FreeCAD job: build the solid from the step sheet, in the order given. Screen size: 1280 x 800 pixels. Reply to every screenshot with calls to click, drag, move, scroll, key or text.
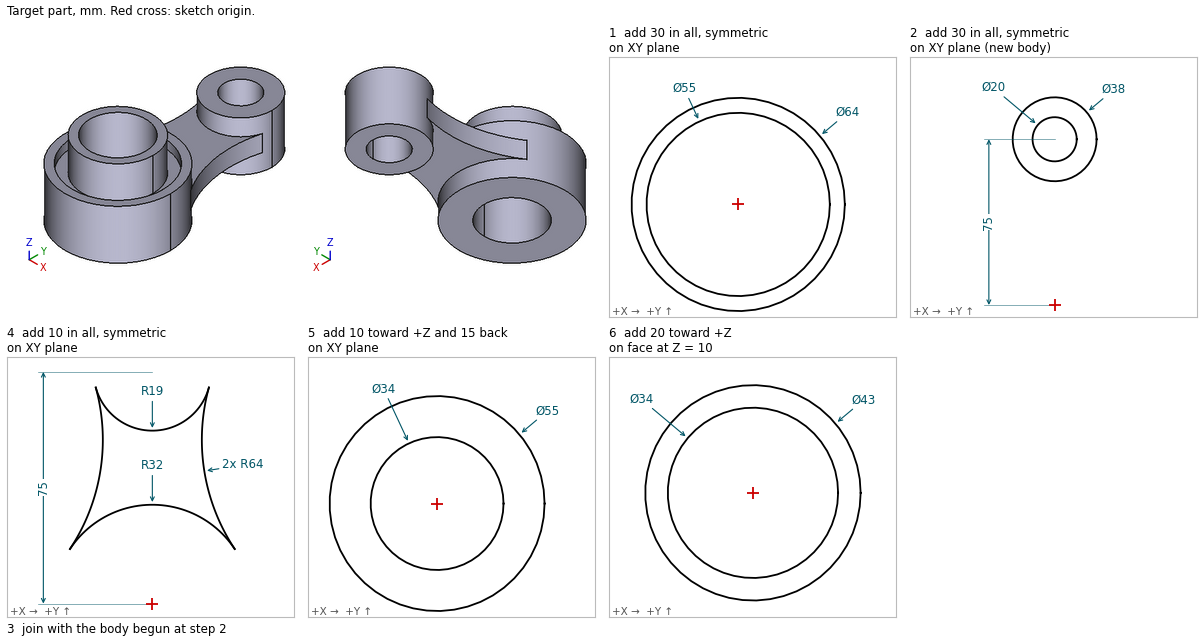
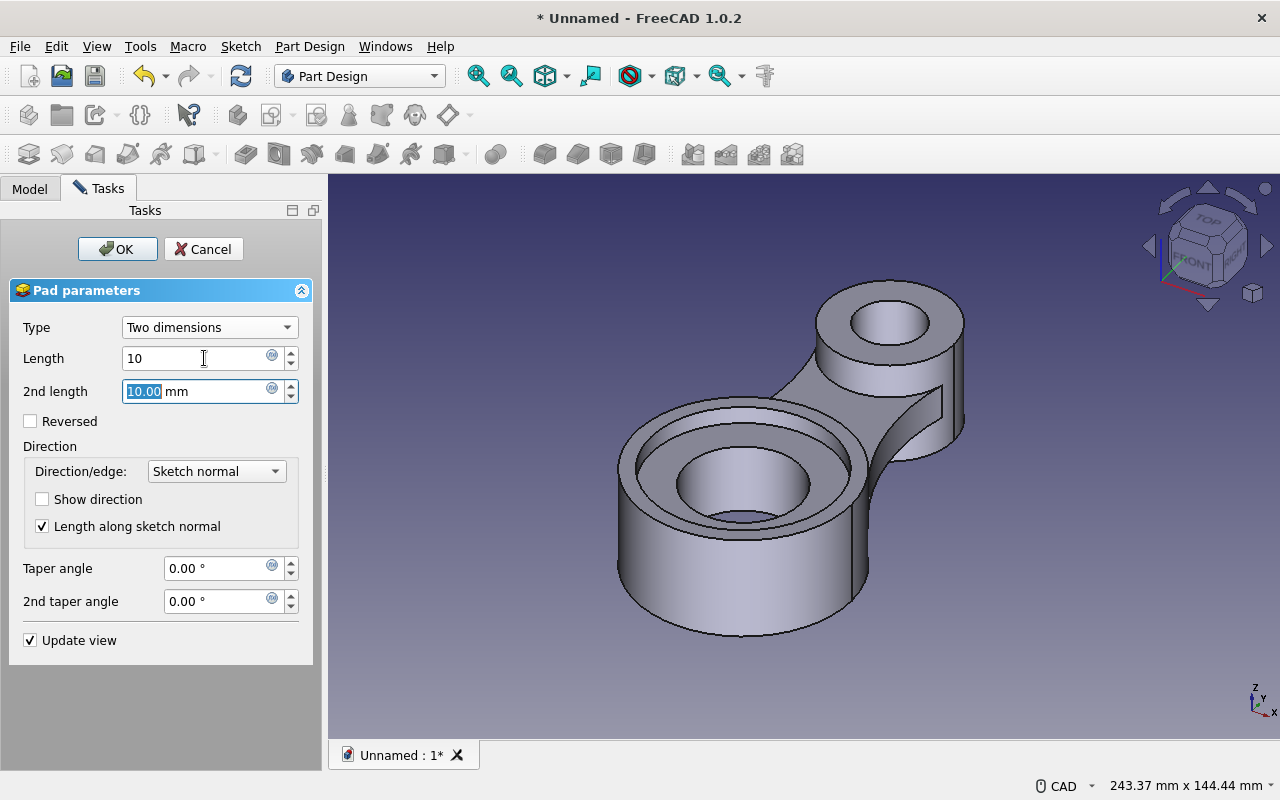
text(15)
key(Tab)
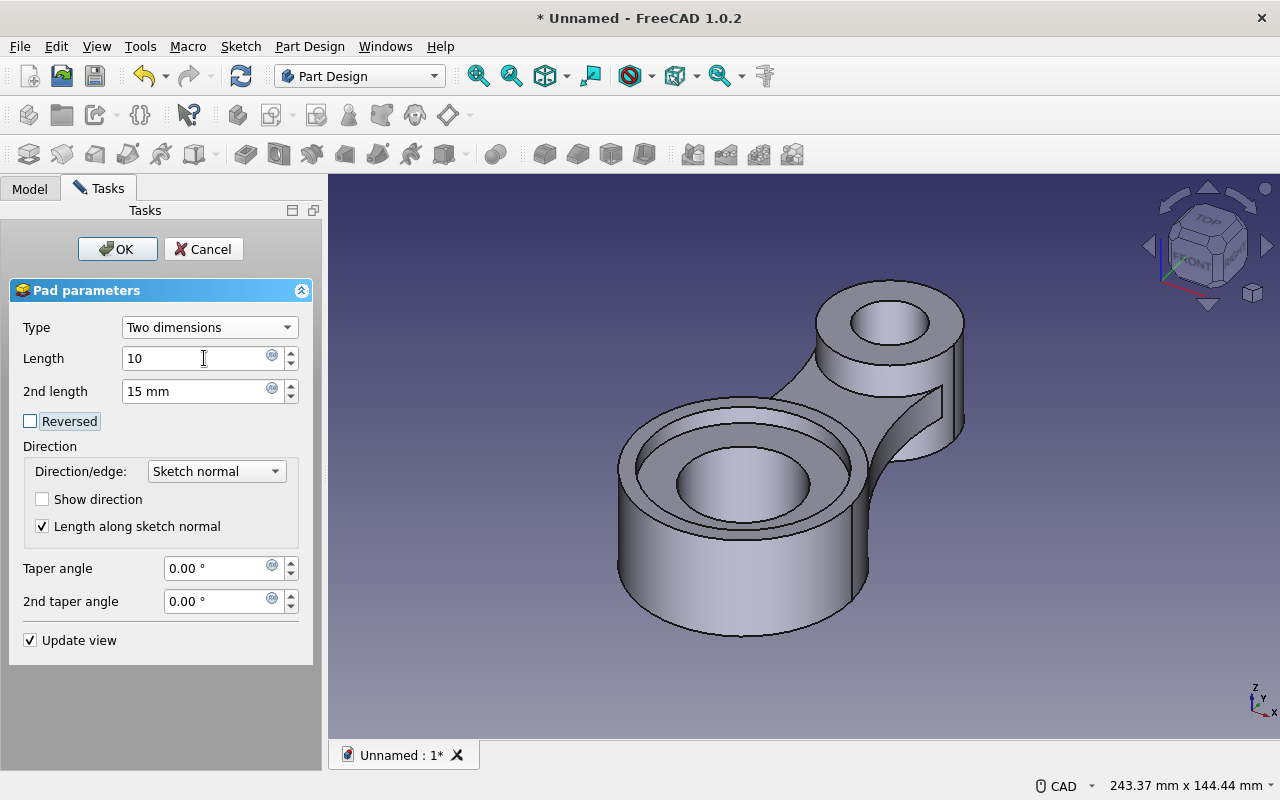
click(118, 249)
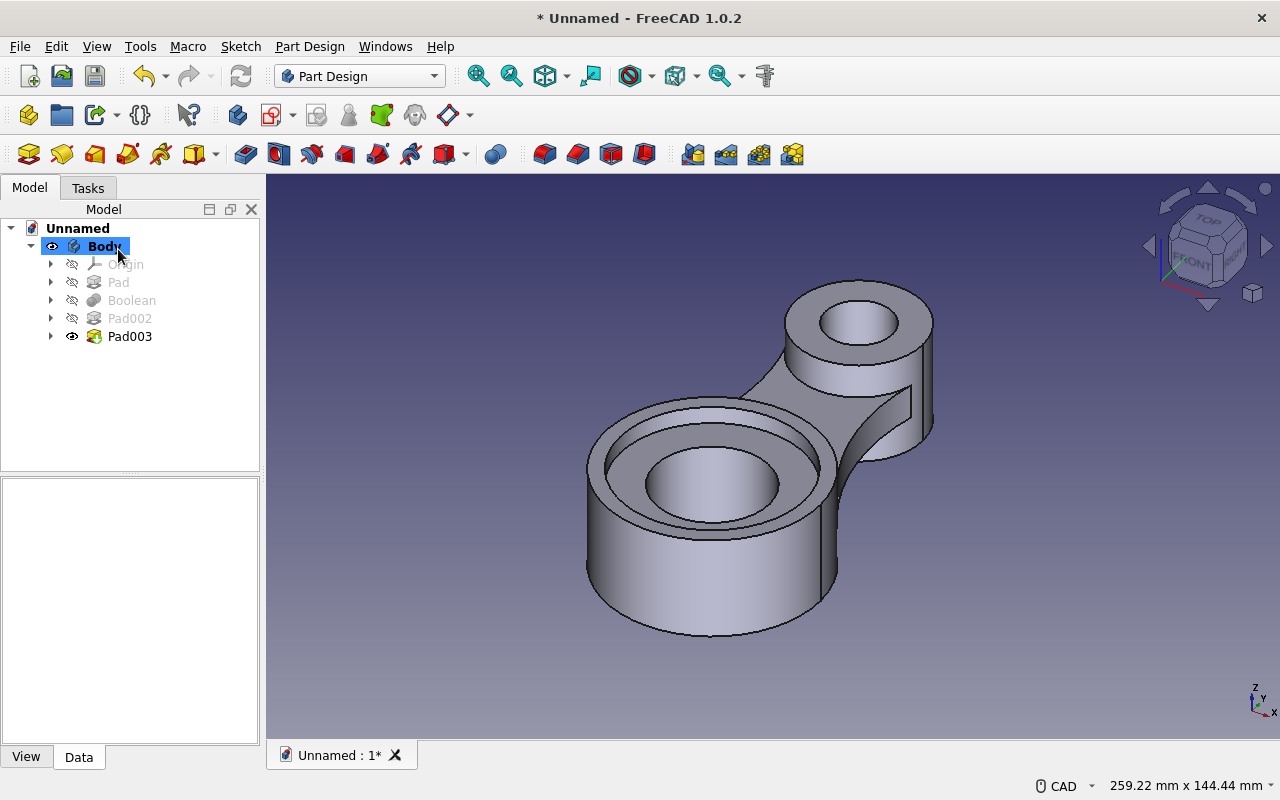
click(690, 436)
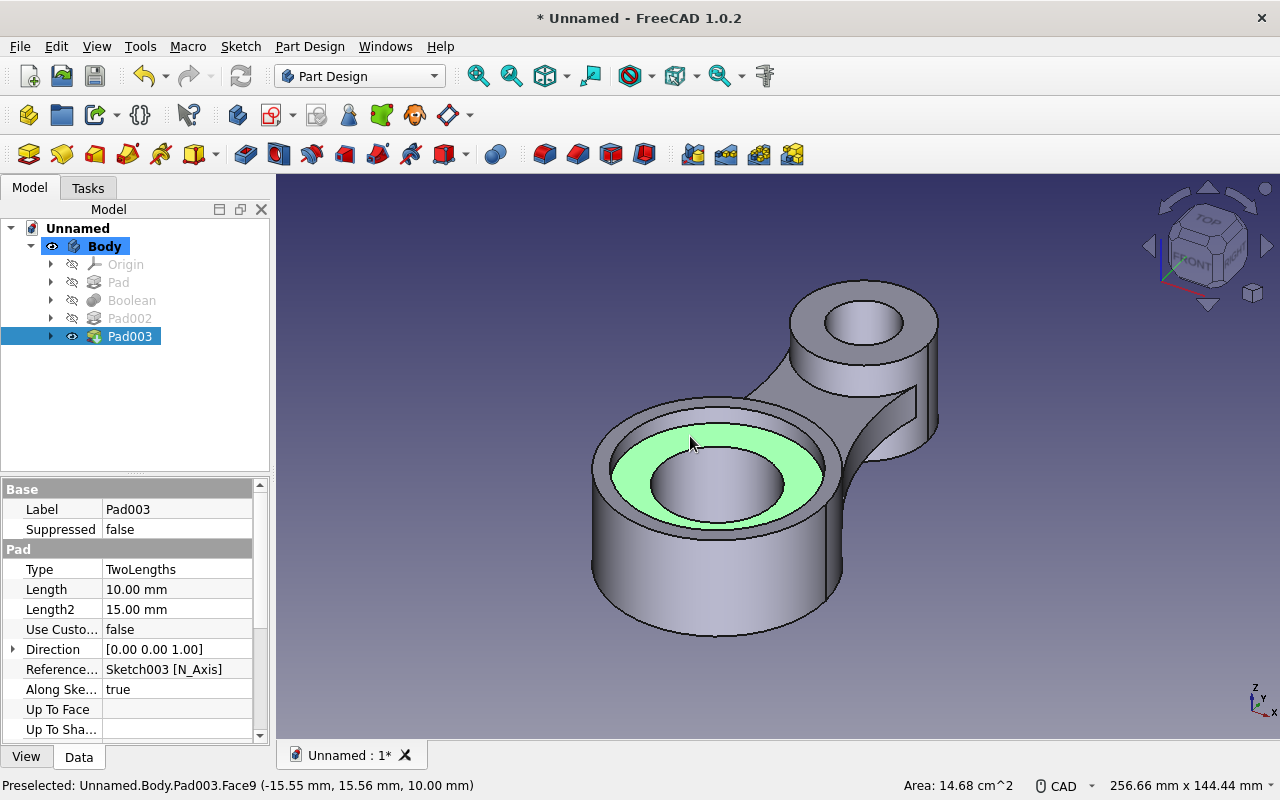
click(270, 116)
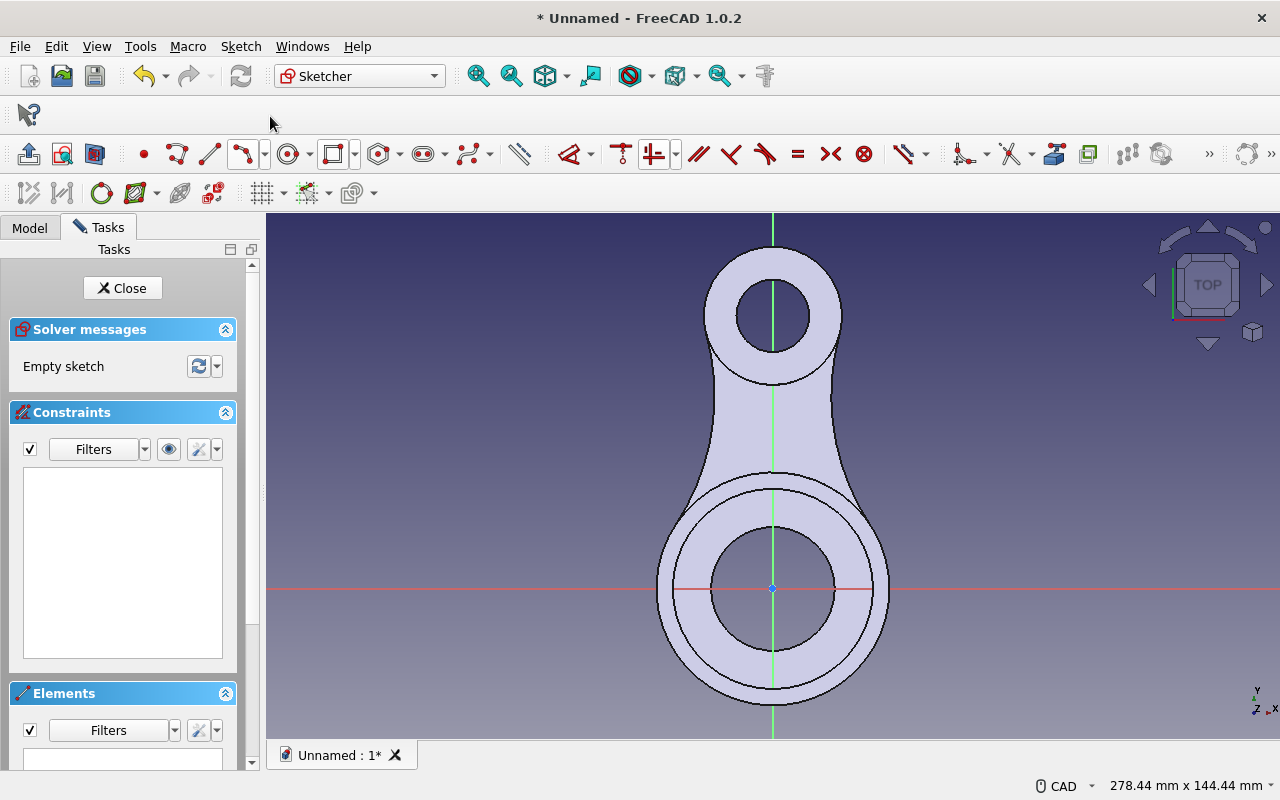
key(q)
key(s)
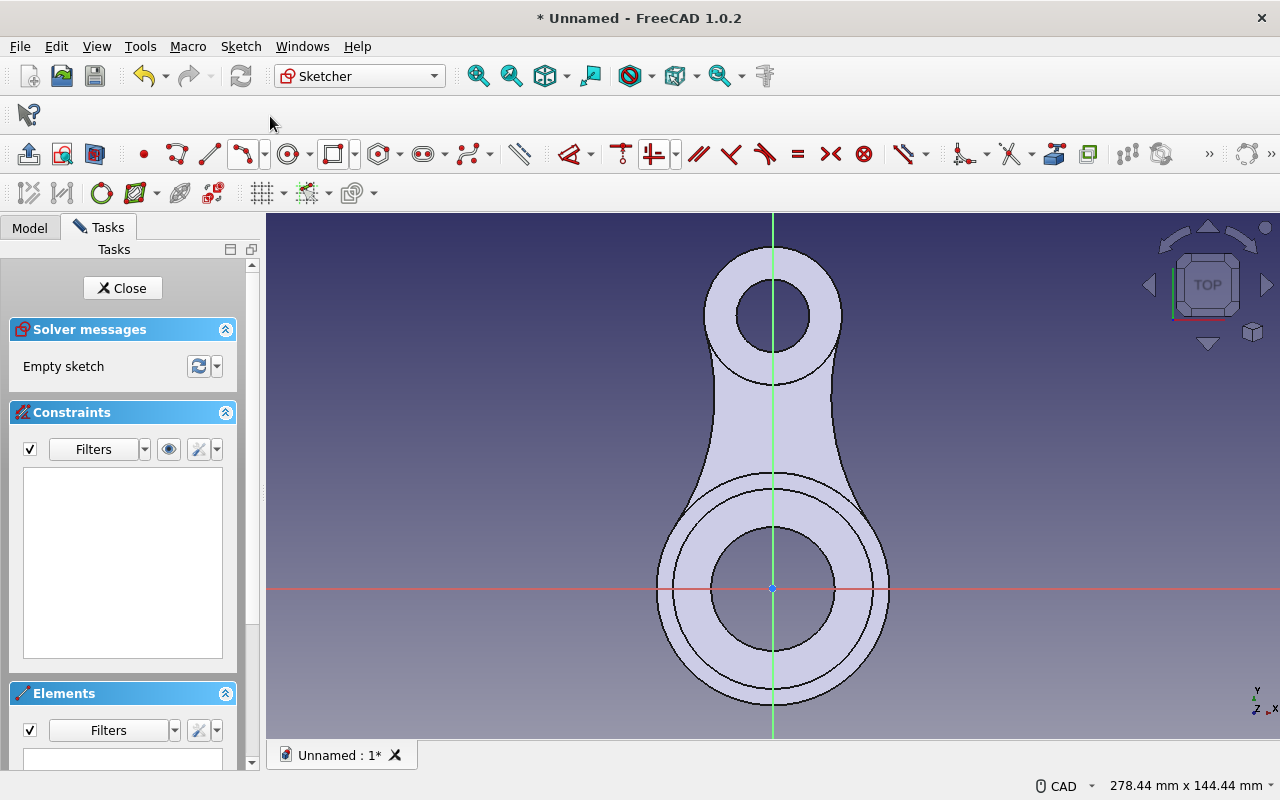
scroll(829, 681, up, 4)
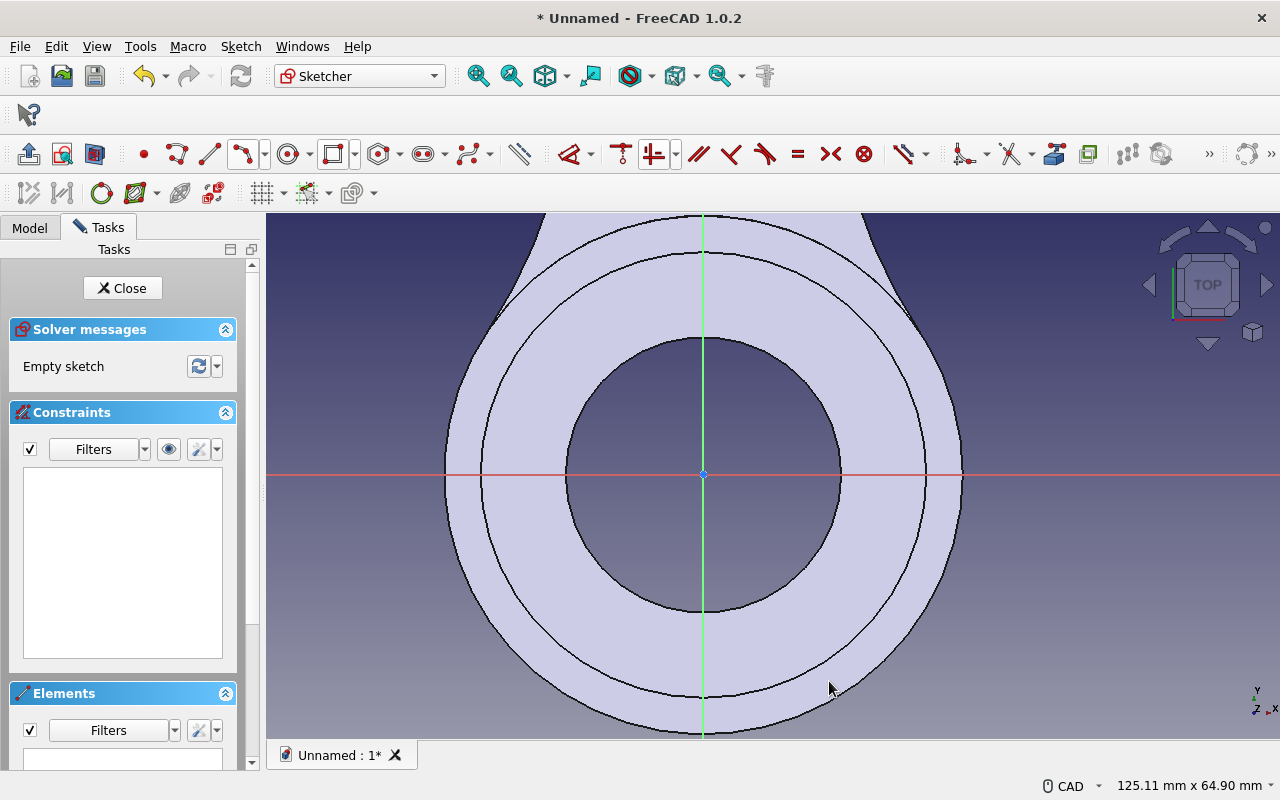
click(288, 154)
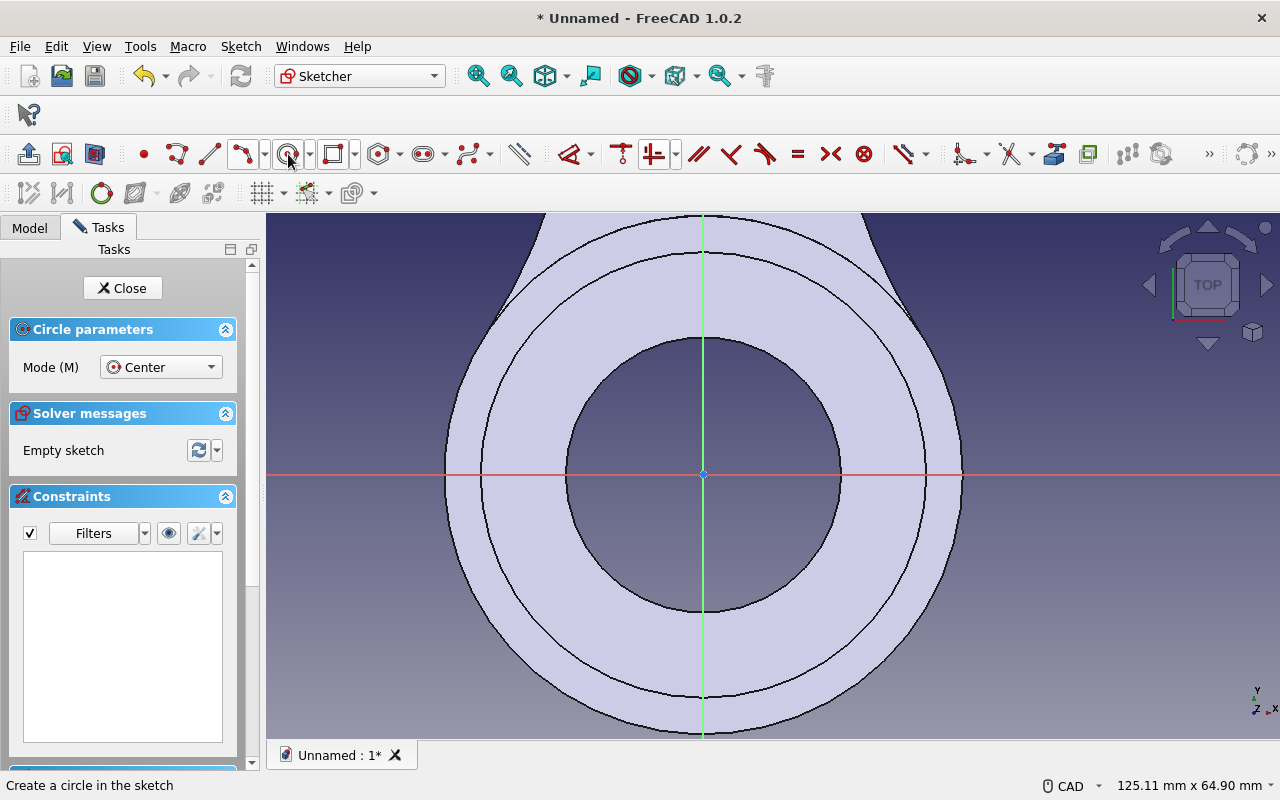
click(703, 475)
click(827, 352)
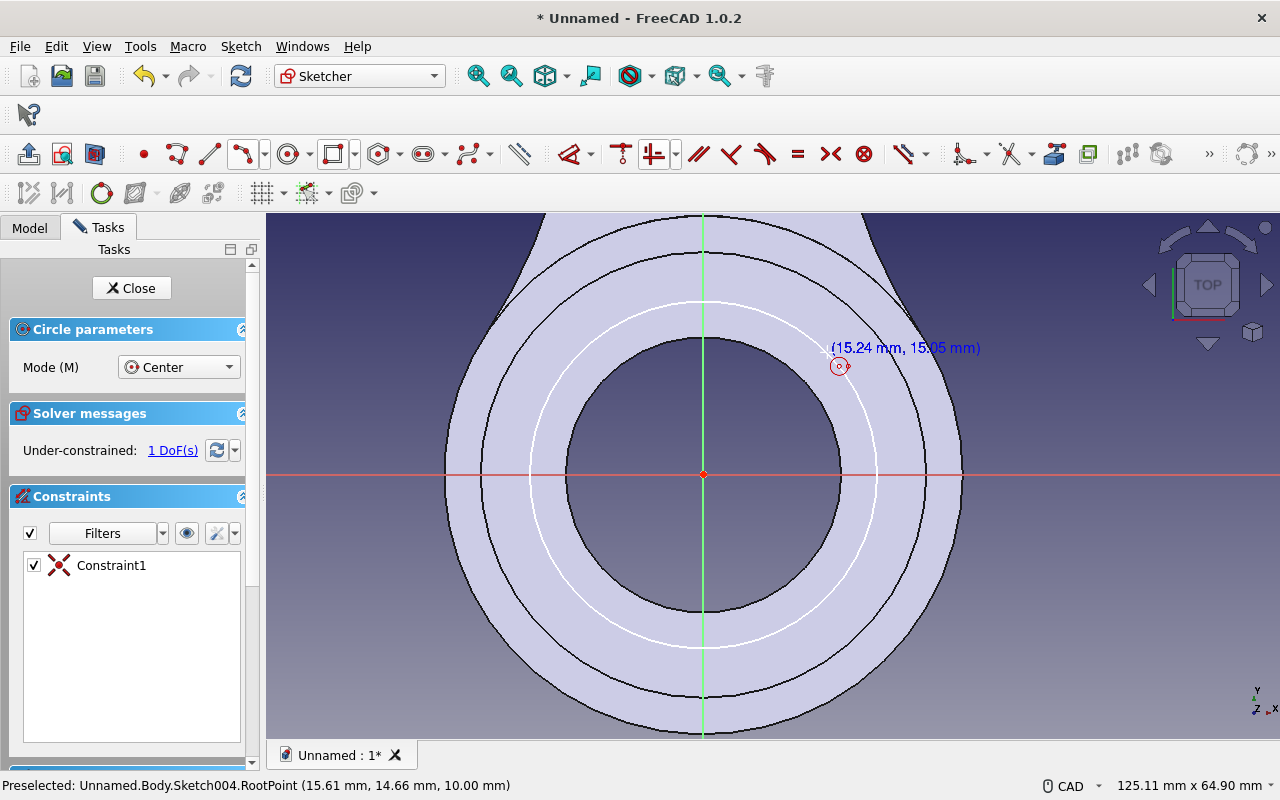
click(703, 475)
click(801, 378)
key(Escape)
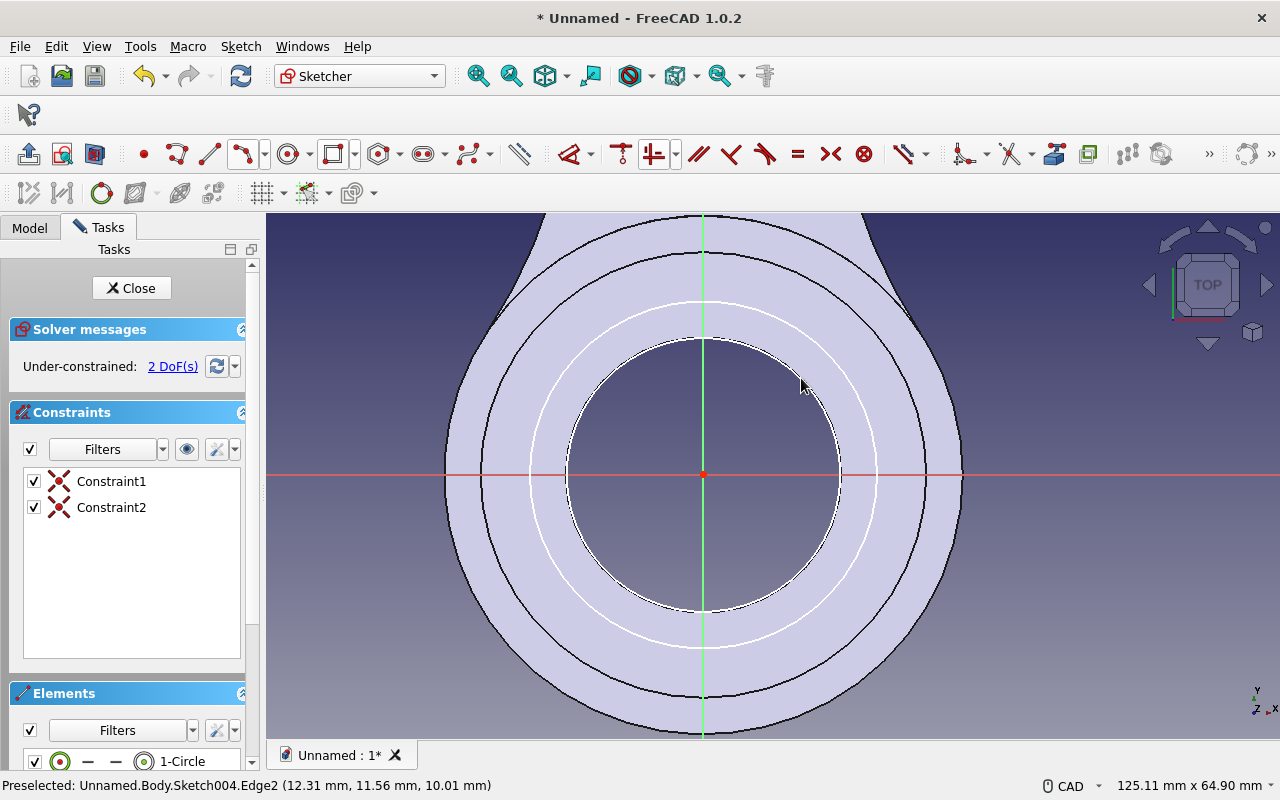
key(d)